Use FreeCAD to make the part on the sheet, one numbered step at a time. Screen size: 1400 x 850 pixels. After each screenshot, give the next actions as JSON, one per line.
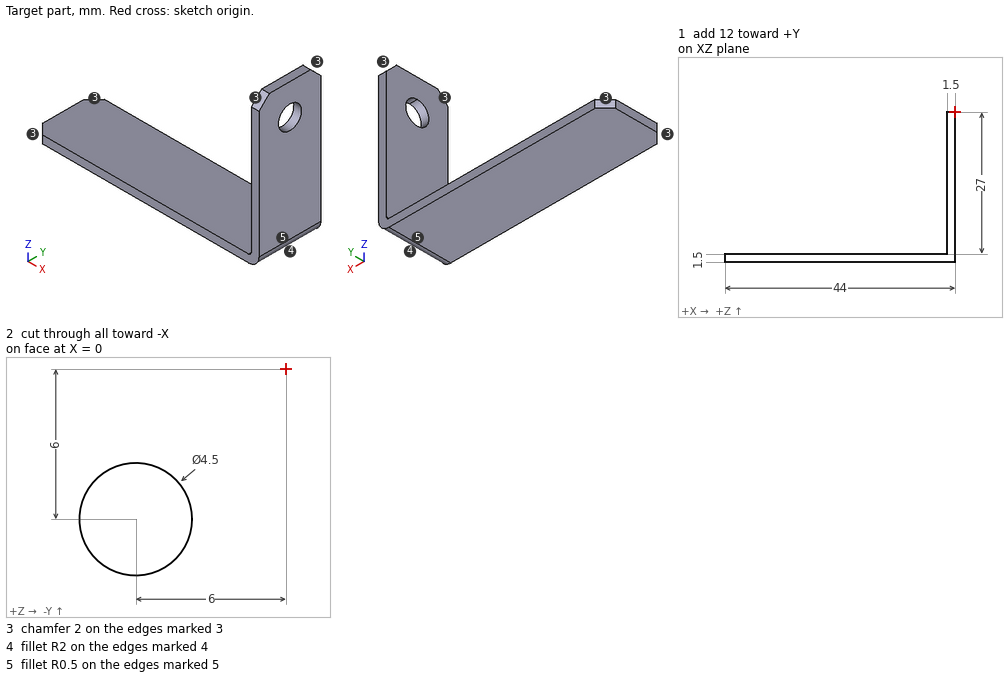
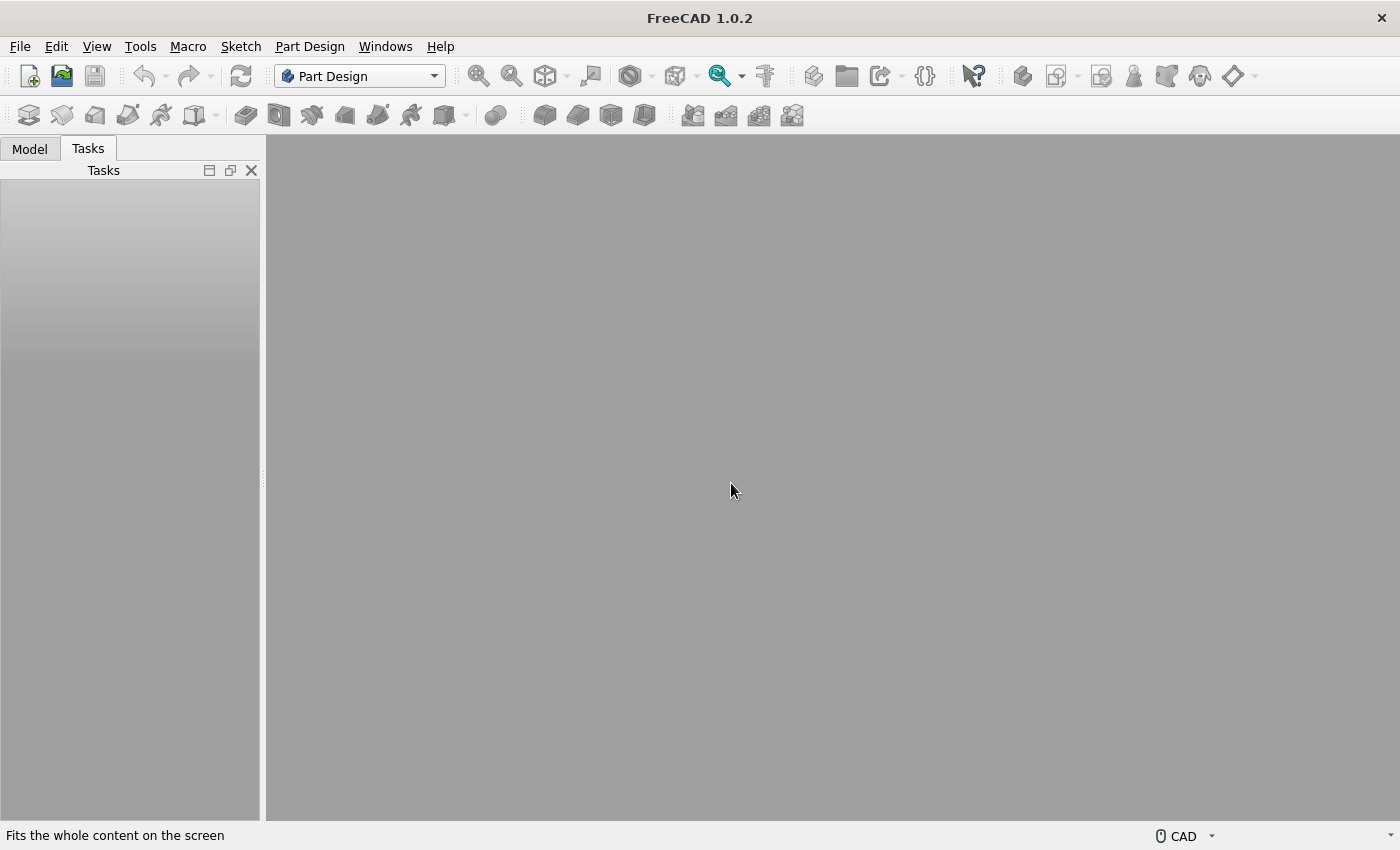
{"action": "key", "text": "ctrl+n"}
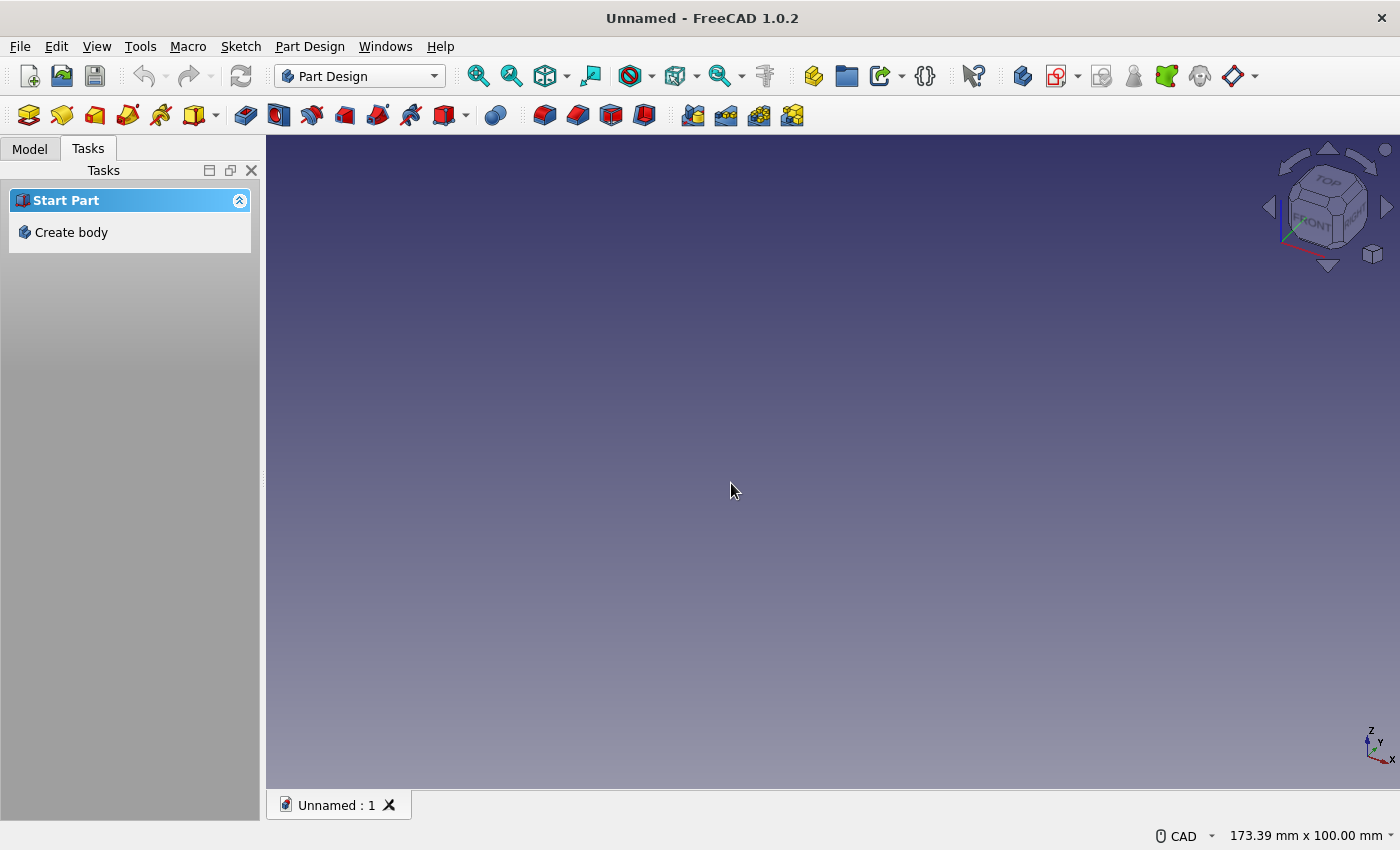
{"action": "left_click", "coordinate": [1056, 76]}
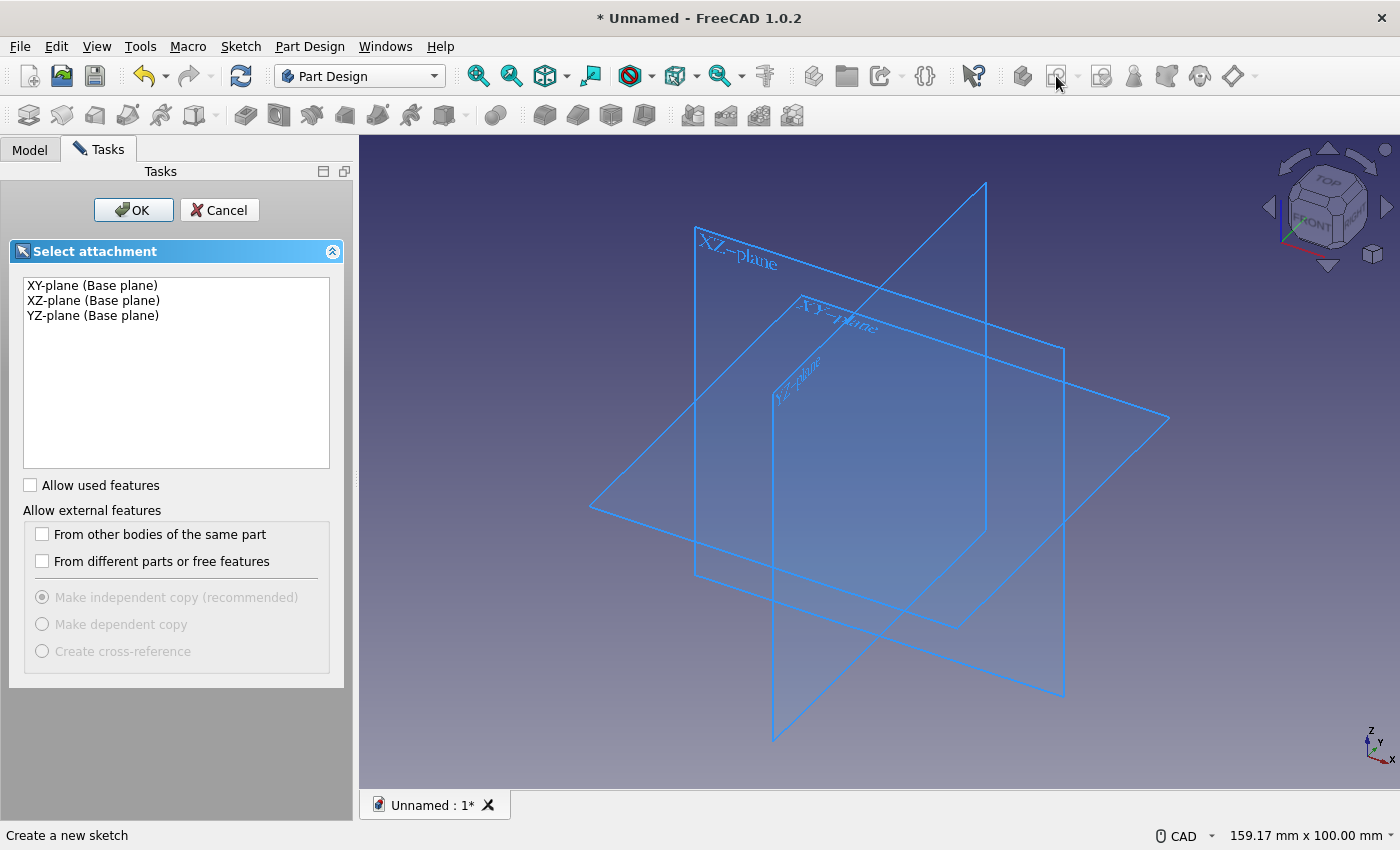
{"action": "left_click", "coordinate": [84, 300]}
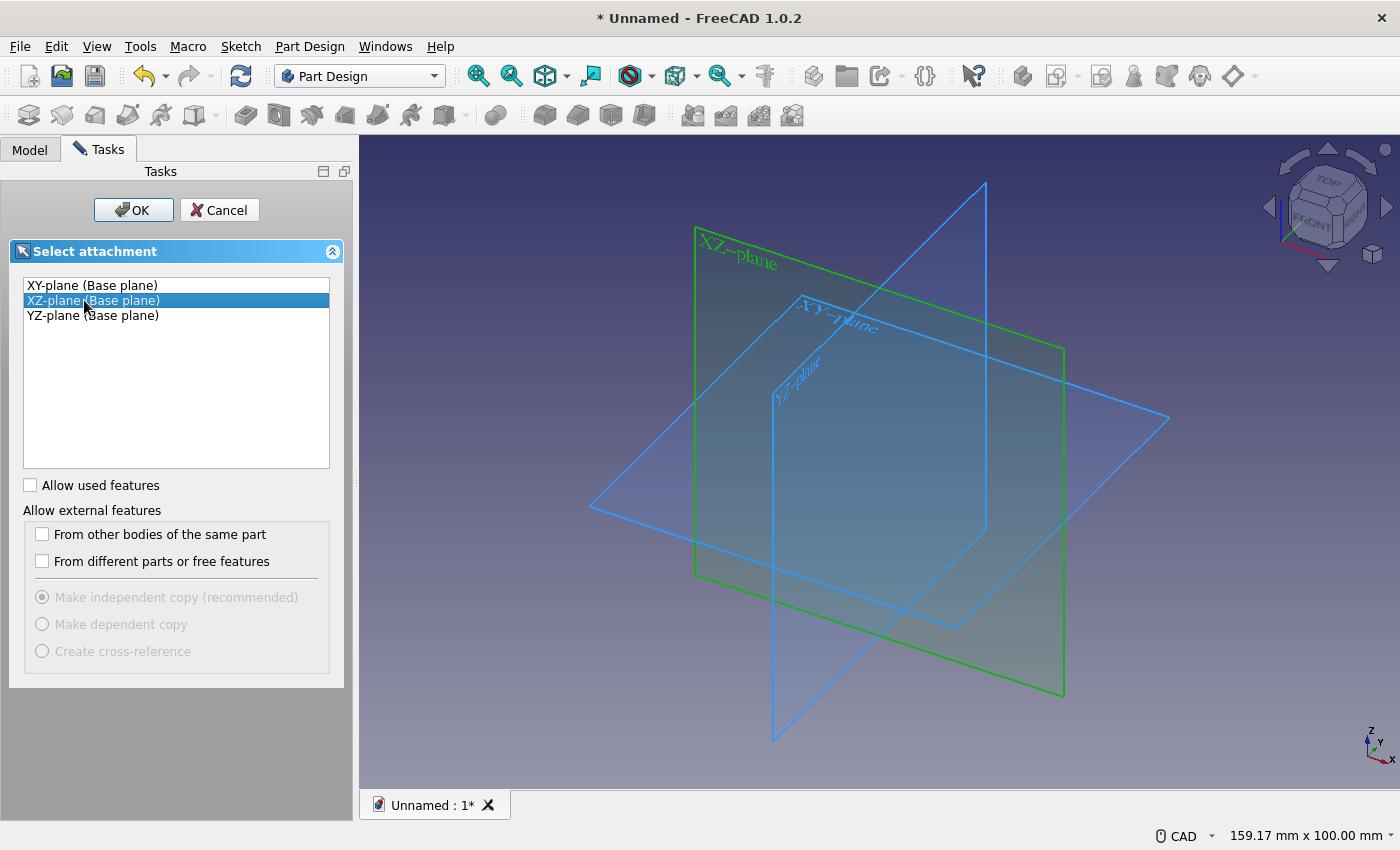
{"action": "left_click", "coordinate": [134, 210]}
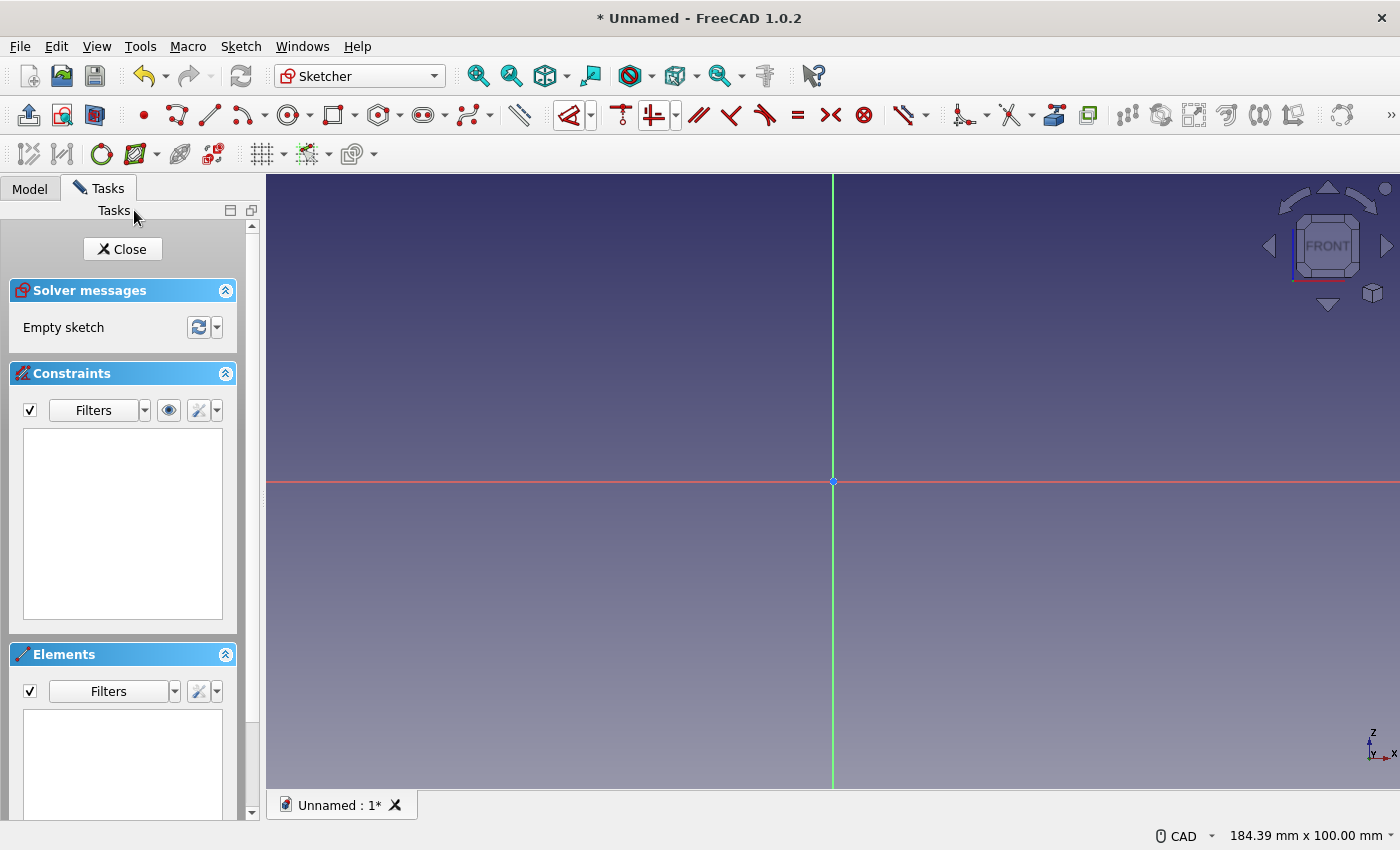
{"action": "scroll", "coordinate": [643, 641], "scroll_direction": "up", "scroll_amount": 4}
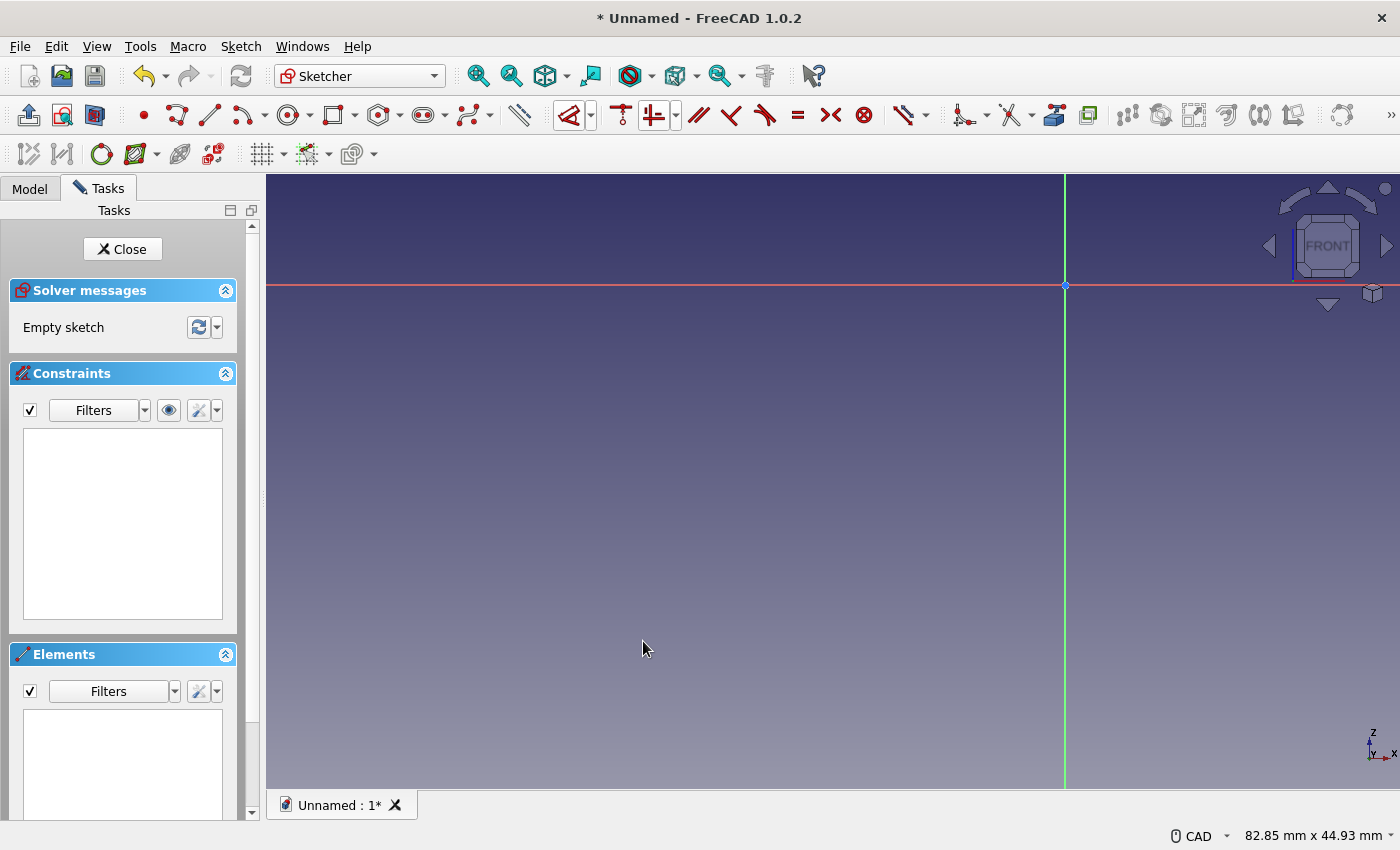
{"action": "left_click", "coordinate": [177, 116]}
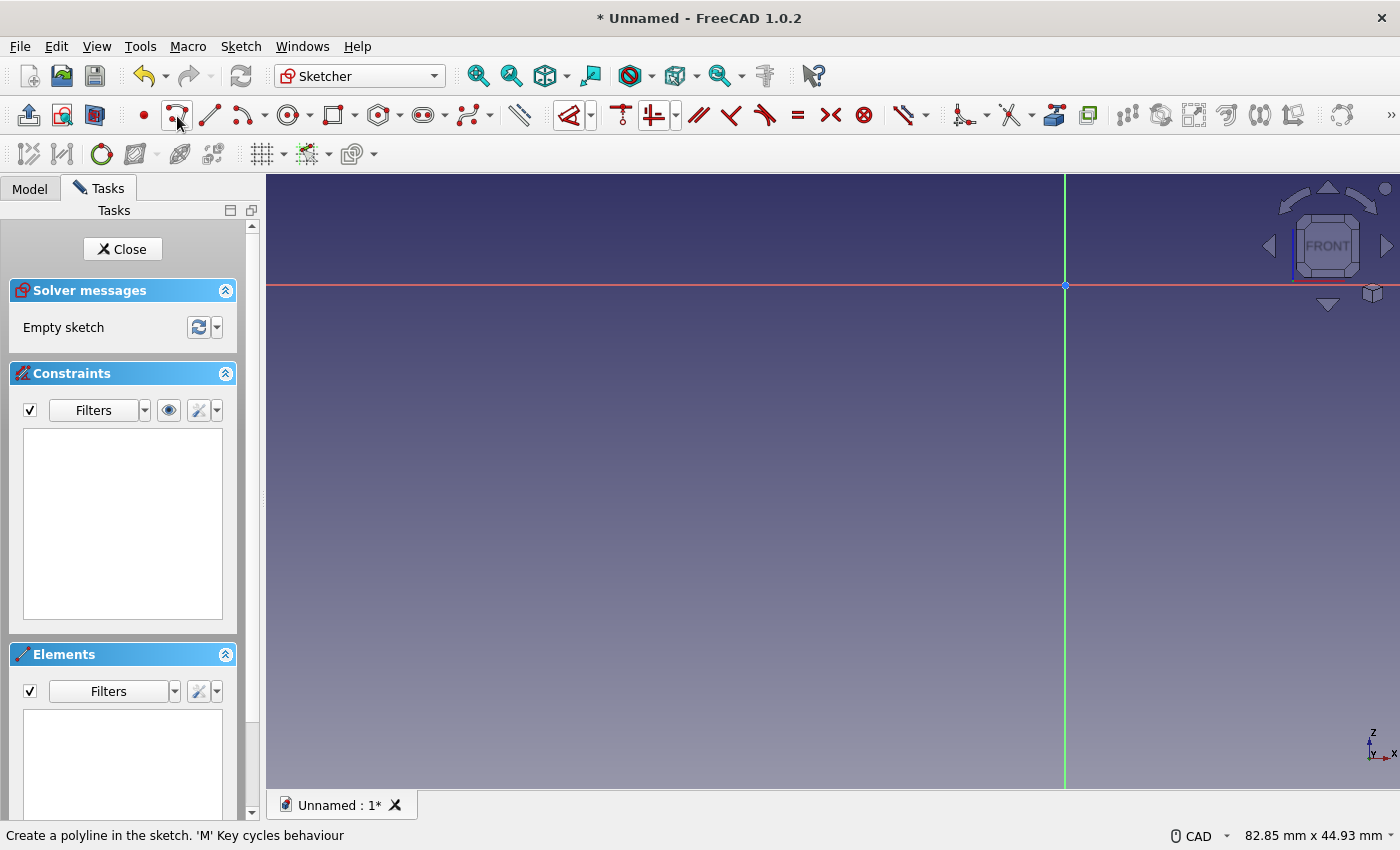
{"action": "left_click", "coordinate": [1065, 285]}
{"action": "left_click", "coordinate": [1056, 675]}
{"action": "left_click", "coordinate": [463, 675]}
{"action": "left_click", "coordinate": [463, 655]}
{"action": "left_click", "coordinate": [1045, 655]}
{"action": "left_click", "coordinate": [1045, 294]}
{"action": "left_click", "coordinate": [1065, 285]}
{"action": "key", "text": "Escape"}
{"action": "key", "text": "Escape"}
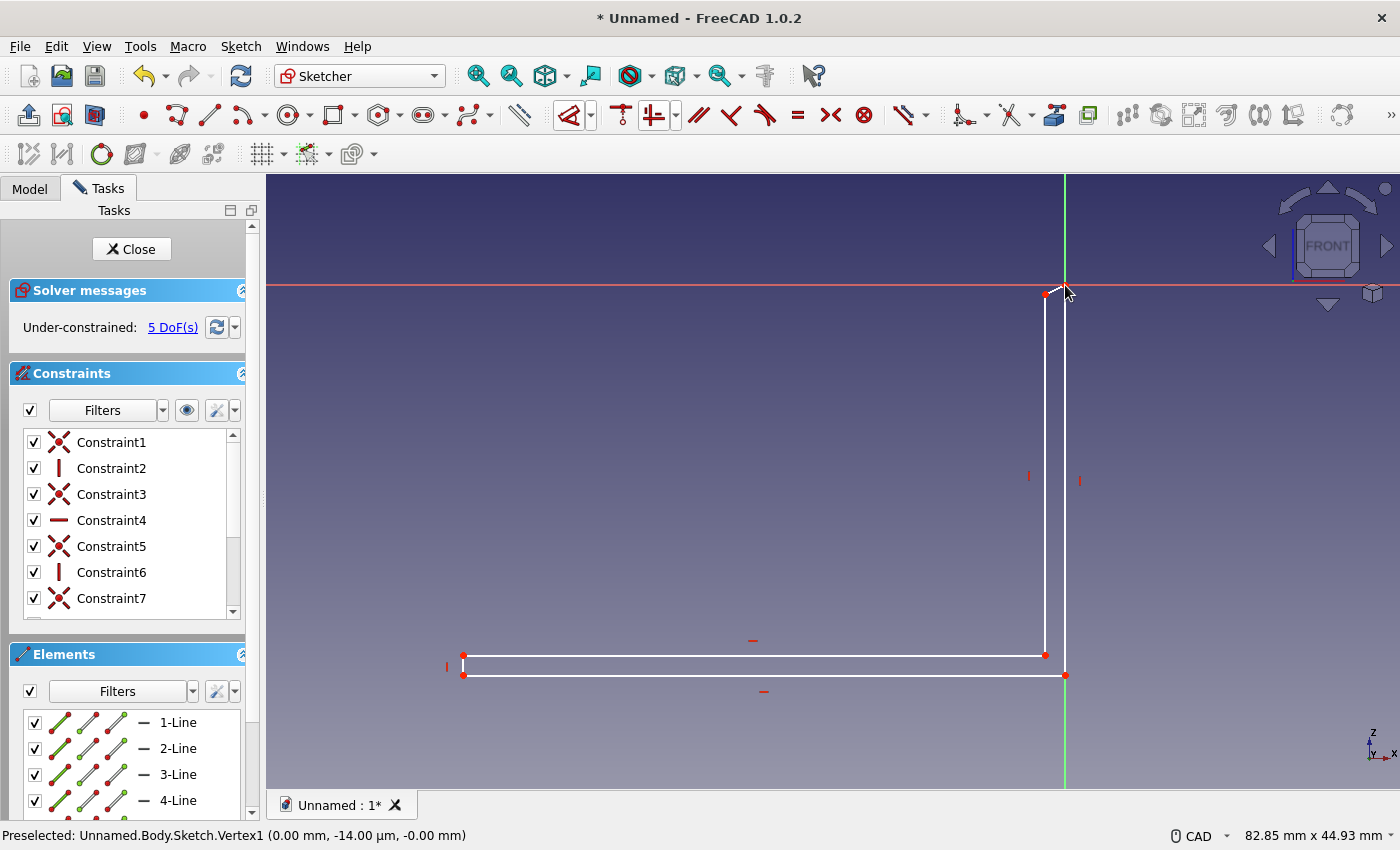
{"action": "scroll", "coordinate": [1057, 289], "scroll_direction": "up", "scroll_amount": 3}